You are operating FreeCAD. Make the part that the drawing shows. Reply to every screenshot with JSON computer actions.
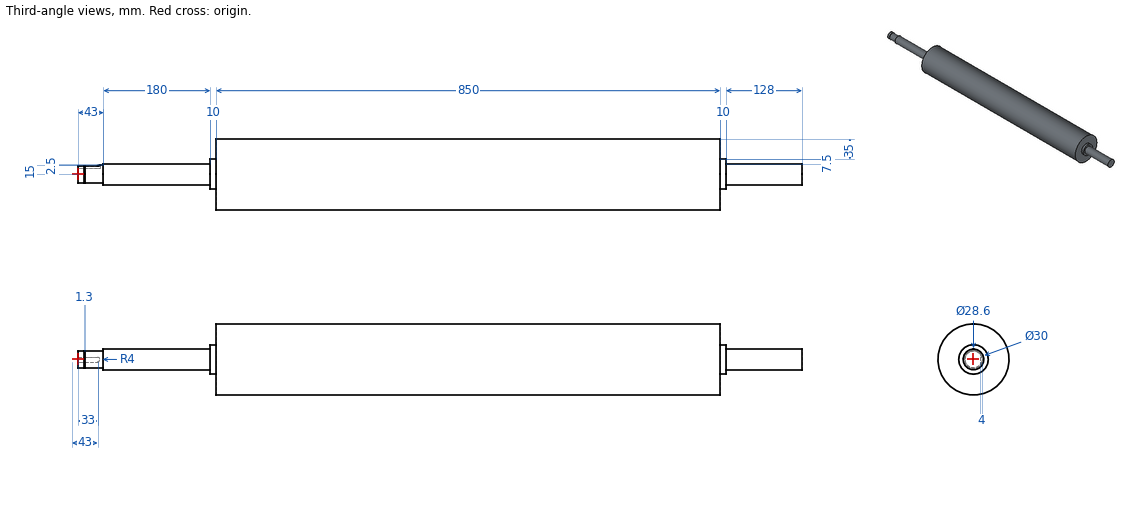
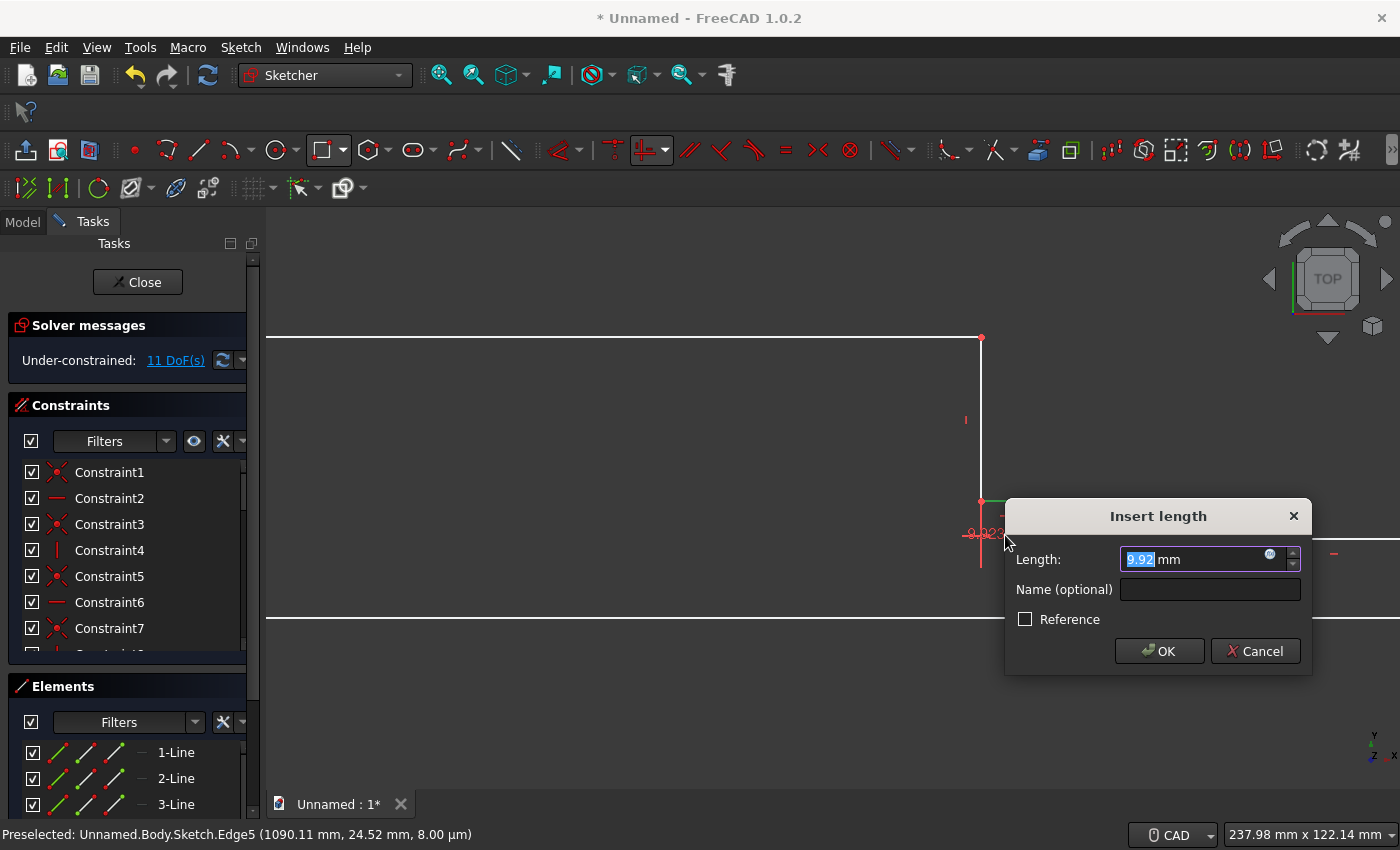
{"action": "type", "text": "10"}
{"action": "key", "text": "Return"}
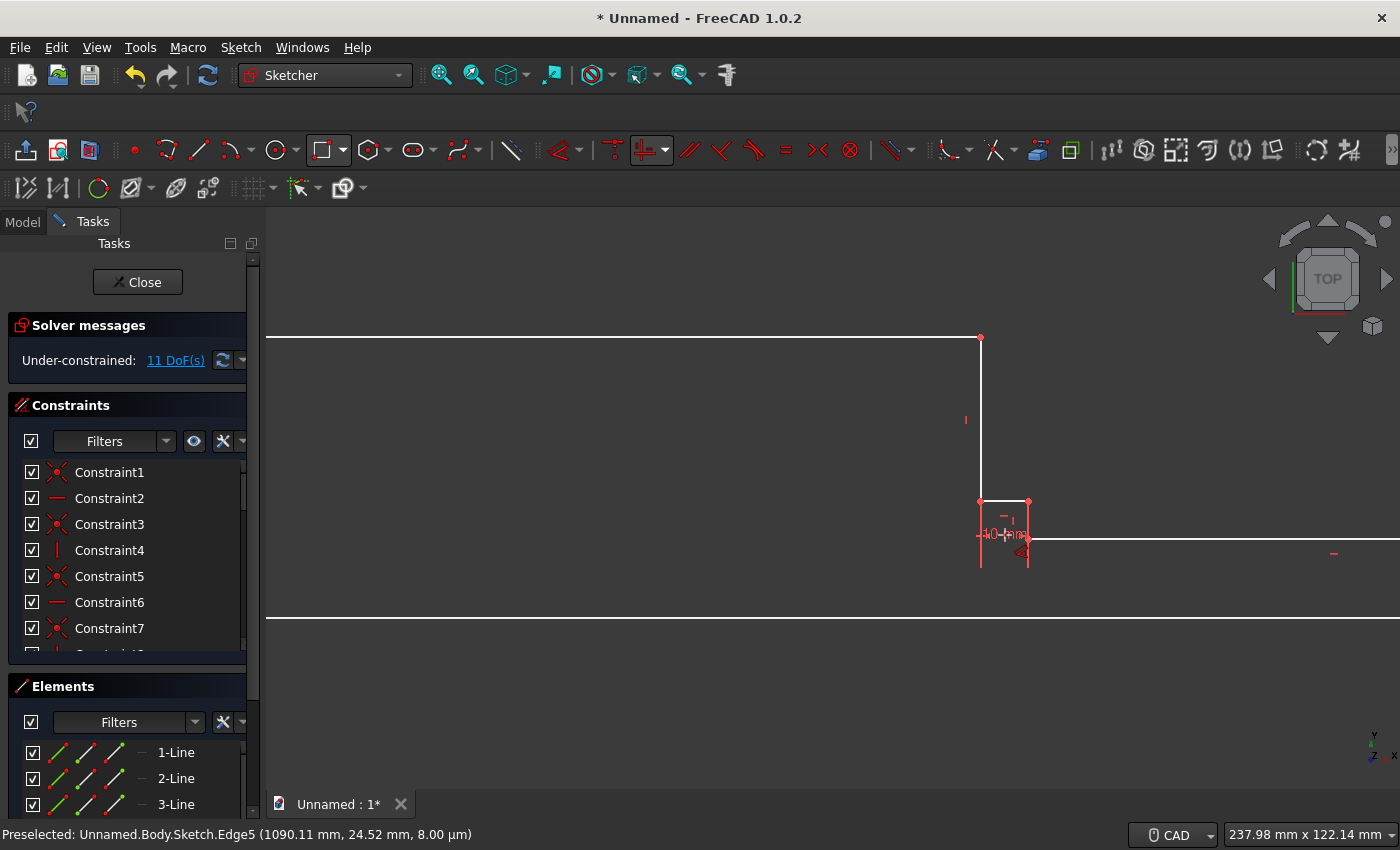
{"action": "scroll", "coordinate": [1018, 501], "scroll_direction": "down", "scroll_amount": 11}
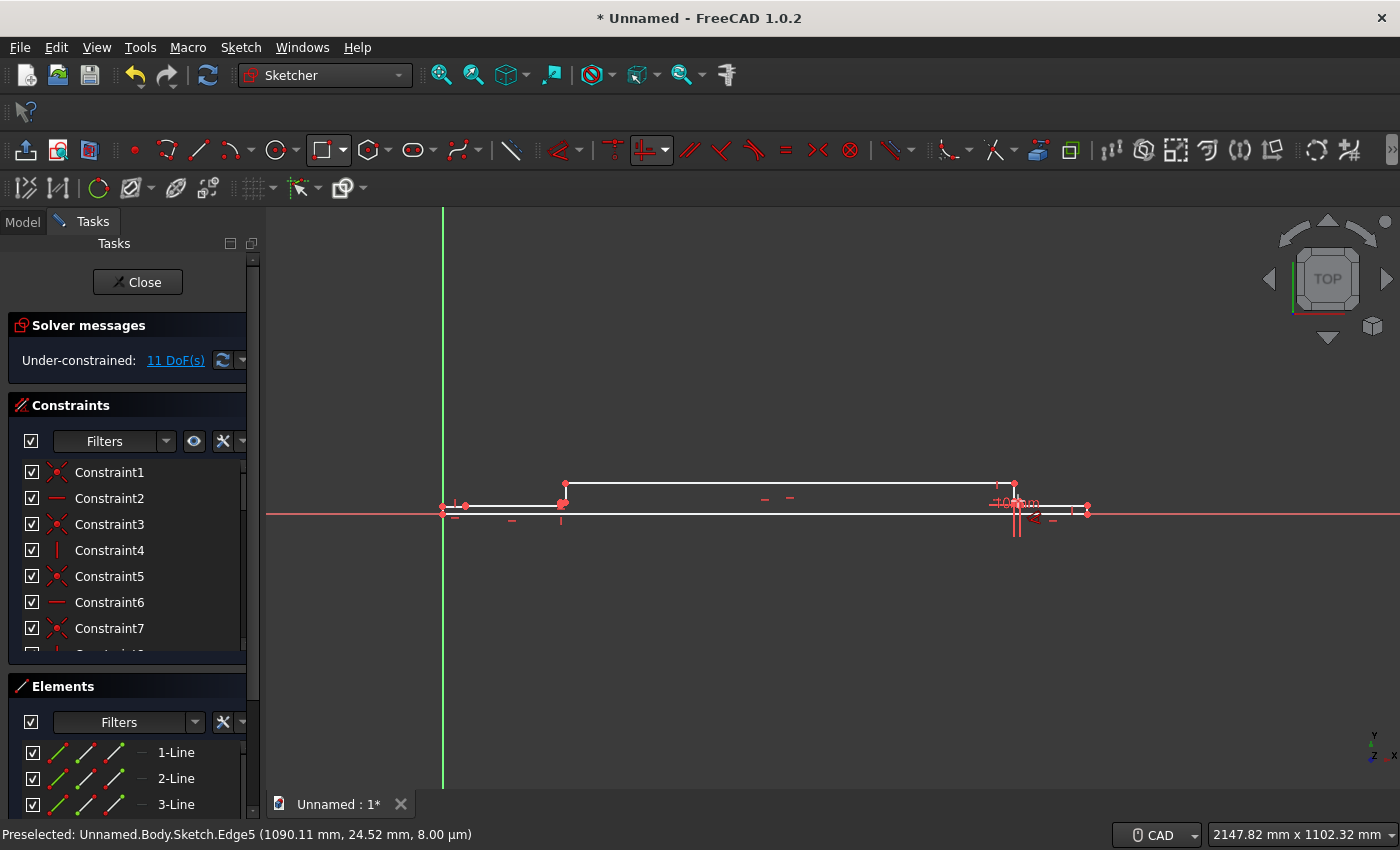
{"action": "scroll", "coordinate": [1014, 496], "scroll_direction": "up", "scroll_amount": 5}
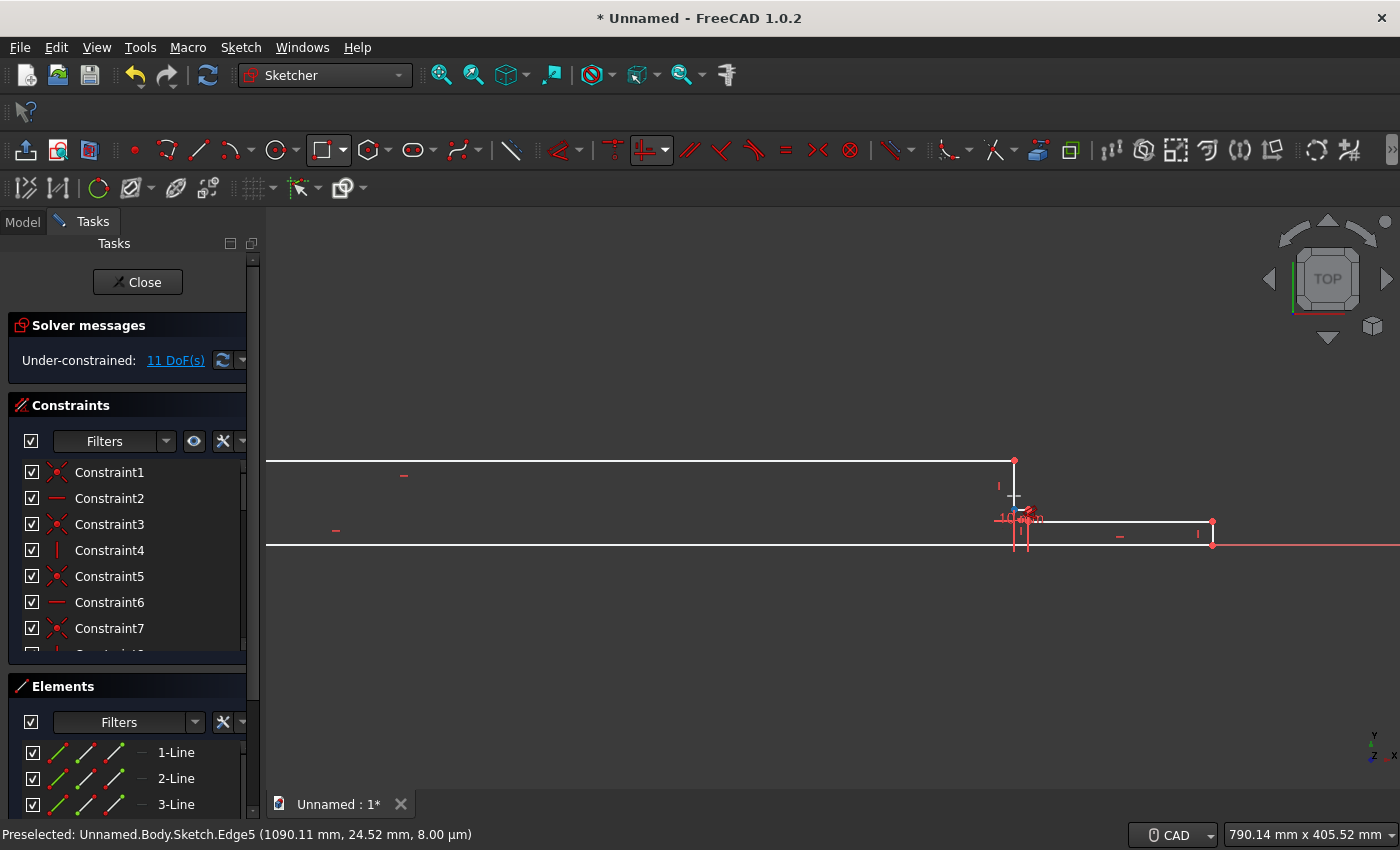
{"action": "left_click", "coordinate": [1014, 495]}
{"action": "left_click", "coordinate": [1048, 485]}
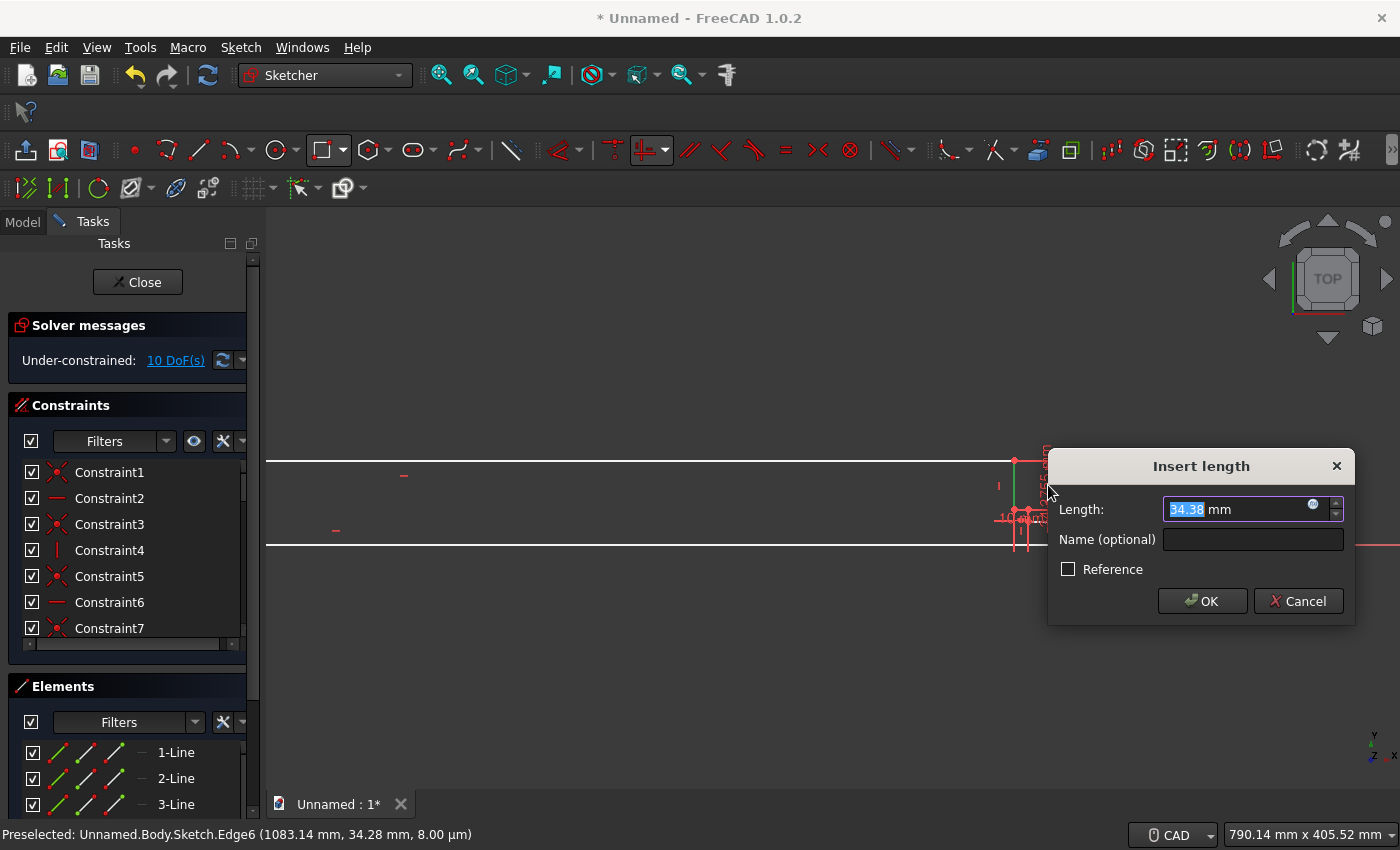
{"action": "type", "text": "35"}
{"action": "key", "text": "Return"}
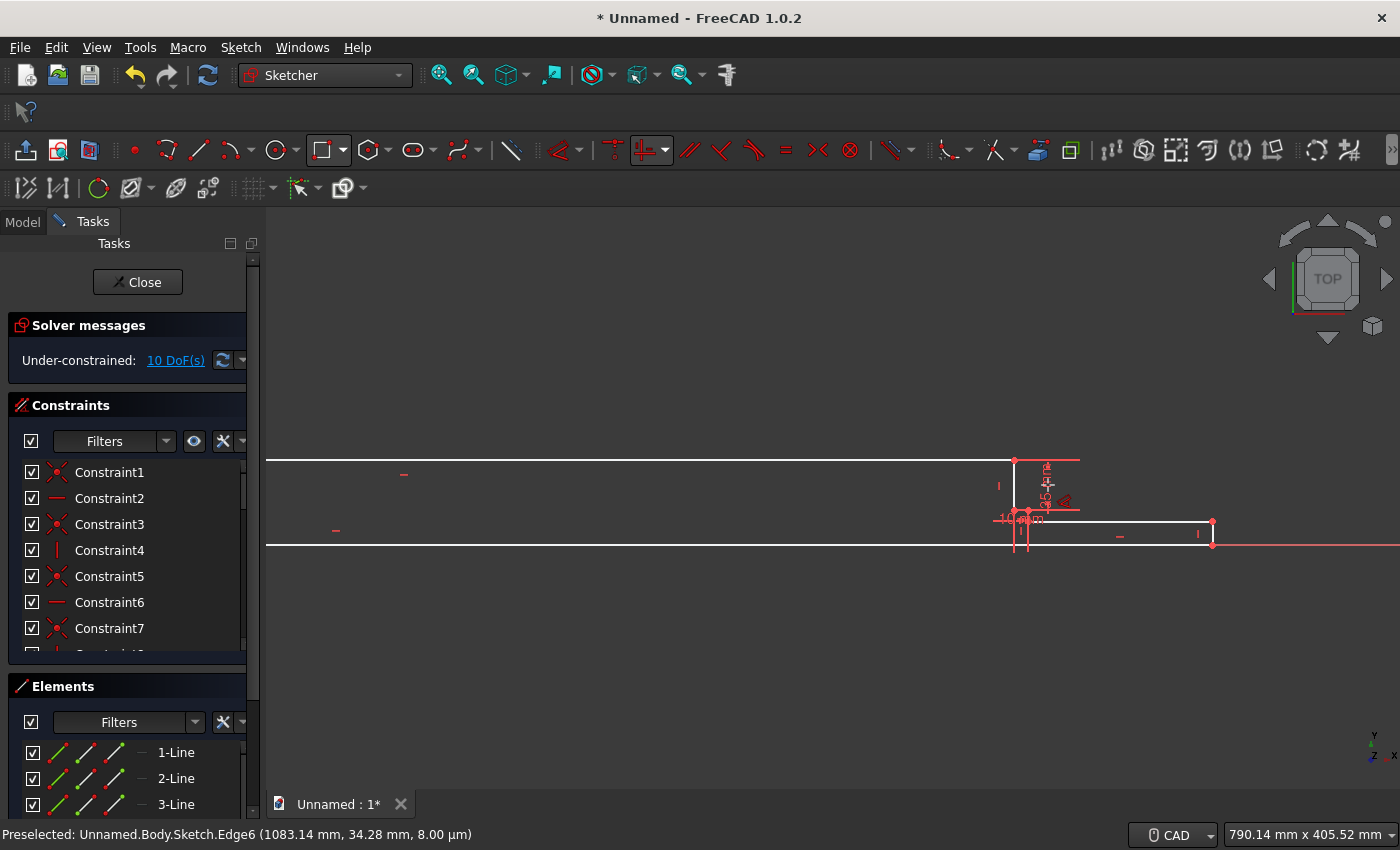
{"action": "scroll", "coordinate": [1014, 496], "scroll_direction": "down", "scroll_amount": 5}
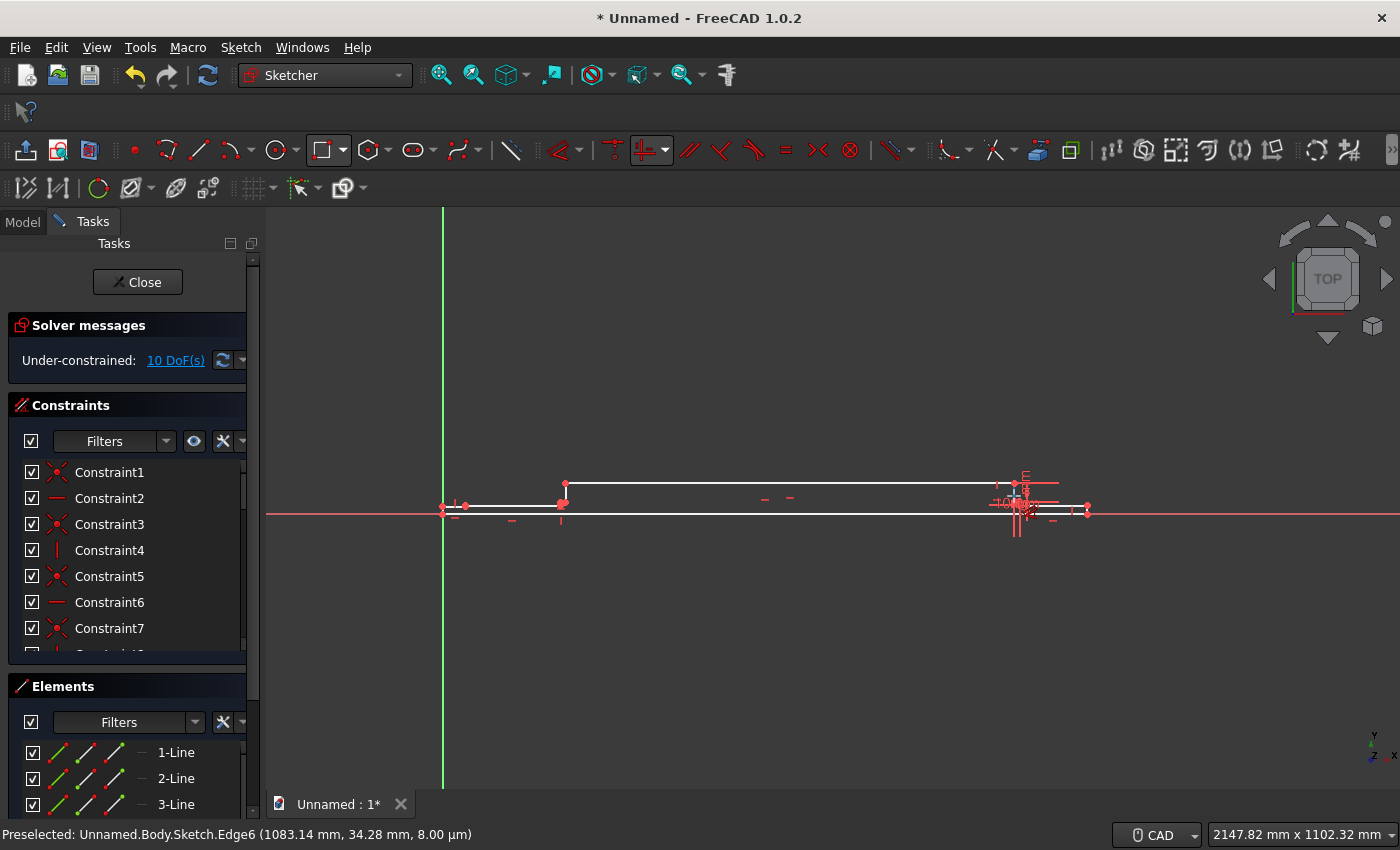
{"action": "scroll", "coordinate": [566, 489], "scroll_direction": "up", "scroll_amount": 5}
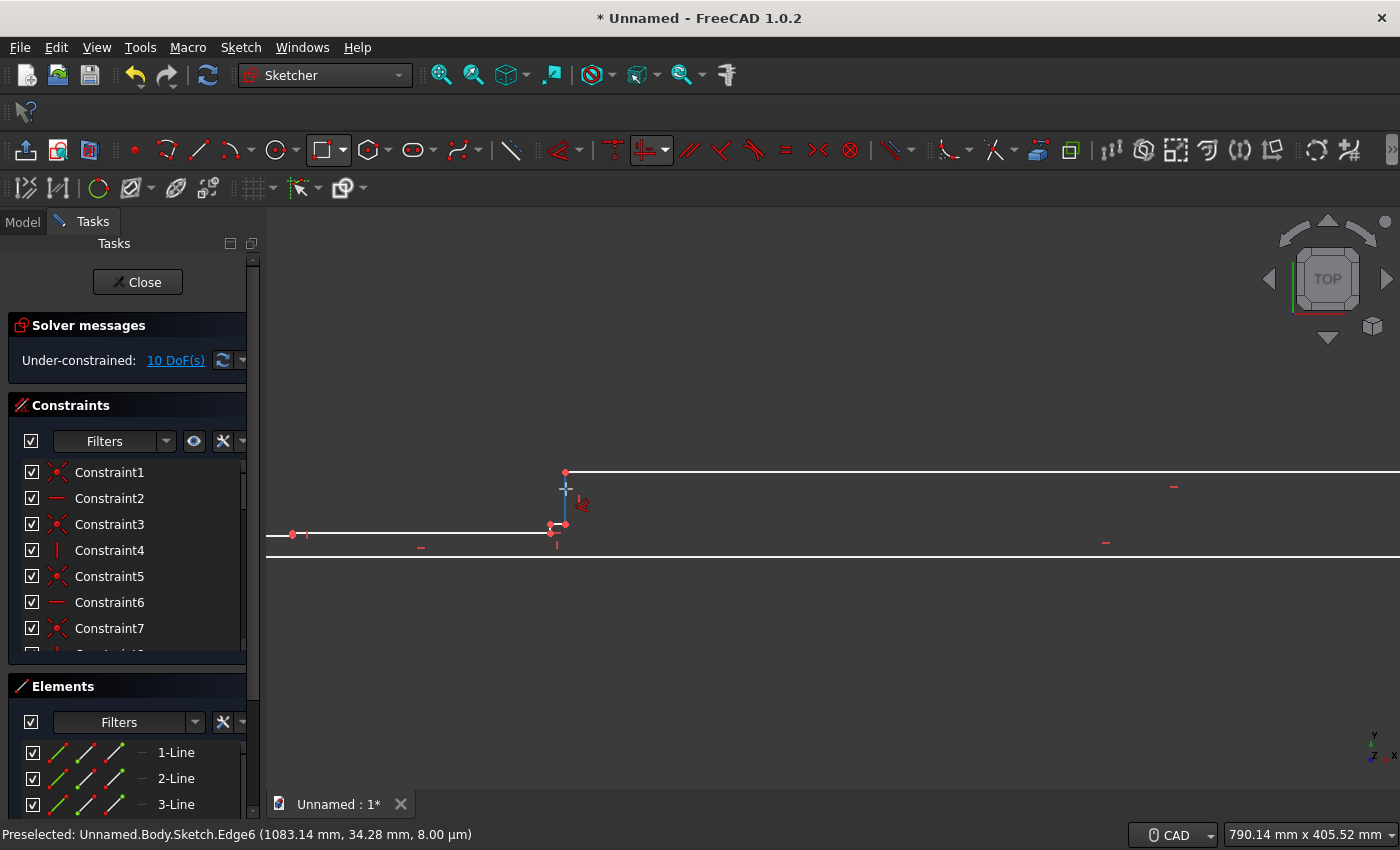
{"action": "left_click", "coordinate": [565, 488]}
{"action": "left_click", "coordinate": [531, 498]}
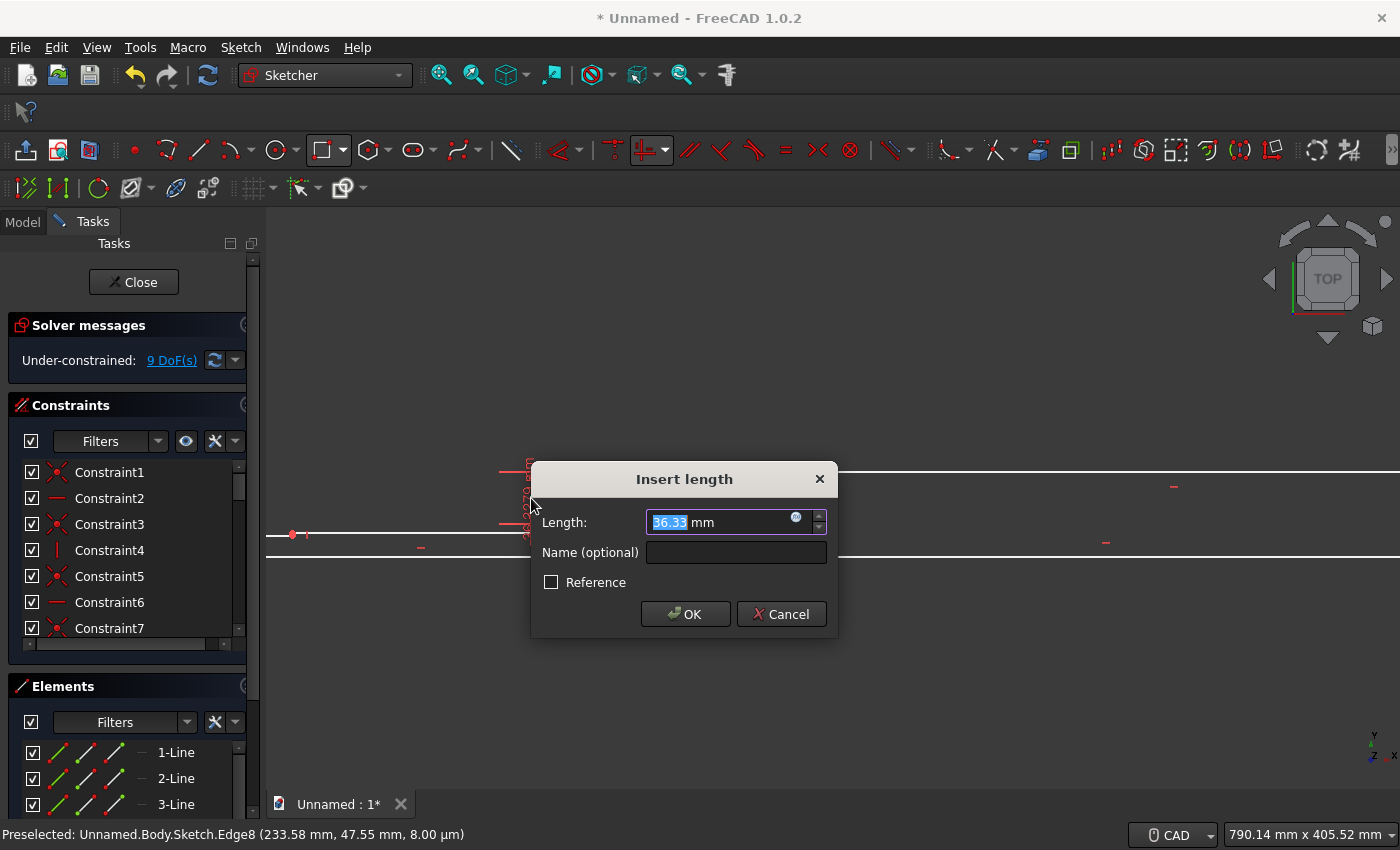
{"action": "type", "text": "35"}
{"action": "key", "text": "Return"}